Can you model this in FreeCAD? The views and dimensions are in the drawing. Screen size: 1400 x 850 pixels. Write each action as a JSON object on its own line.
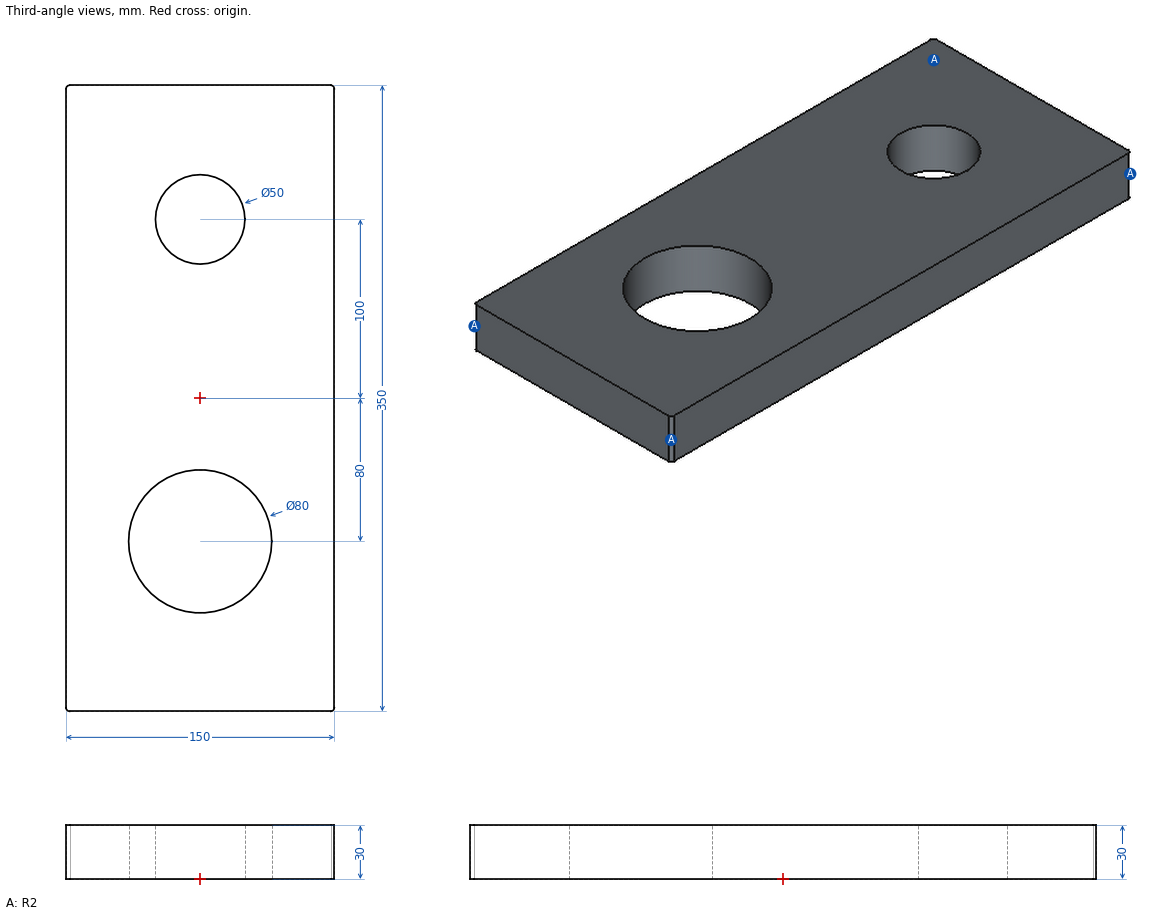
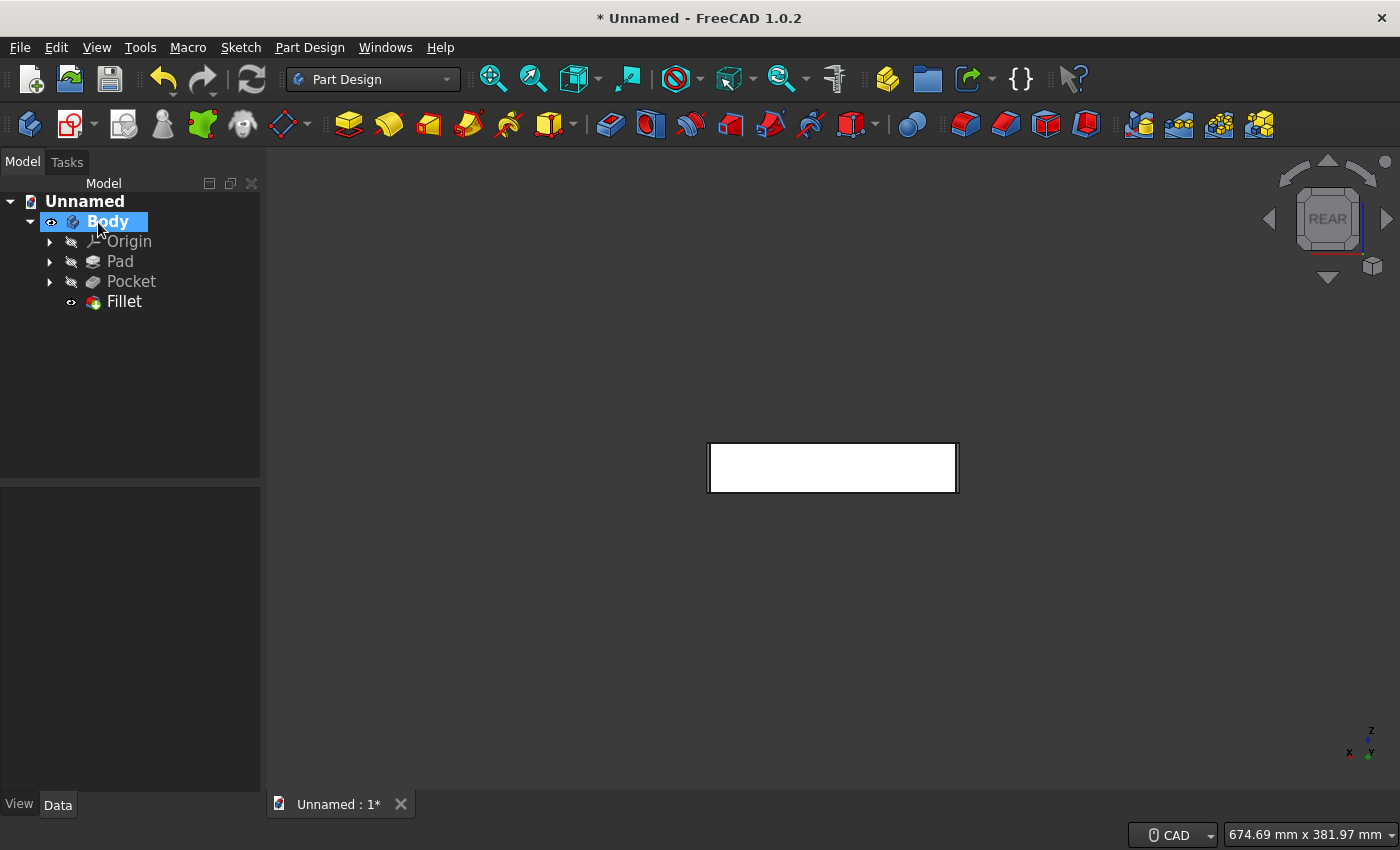
{"action": "key", "text": "0"}